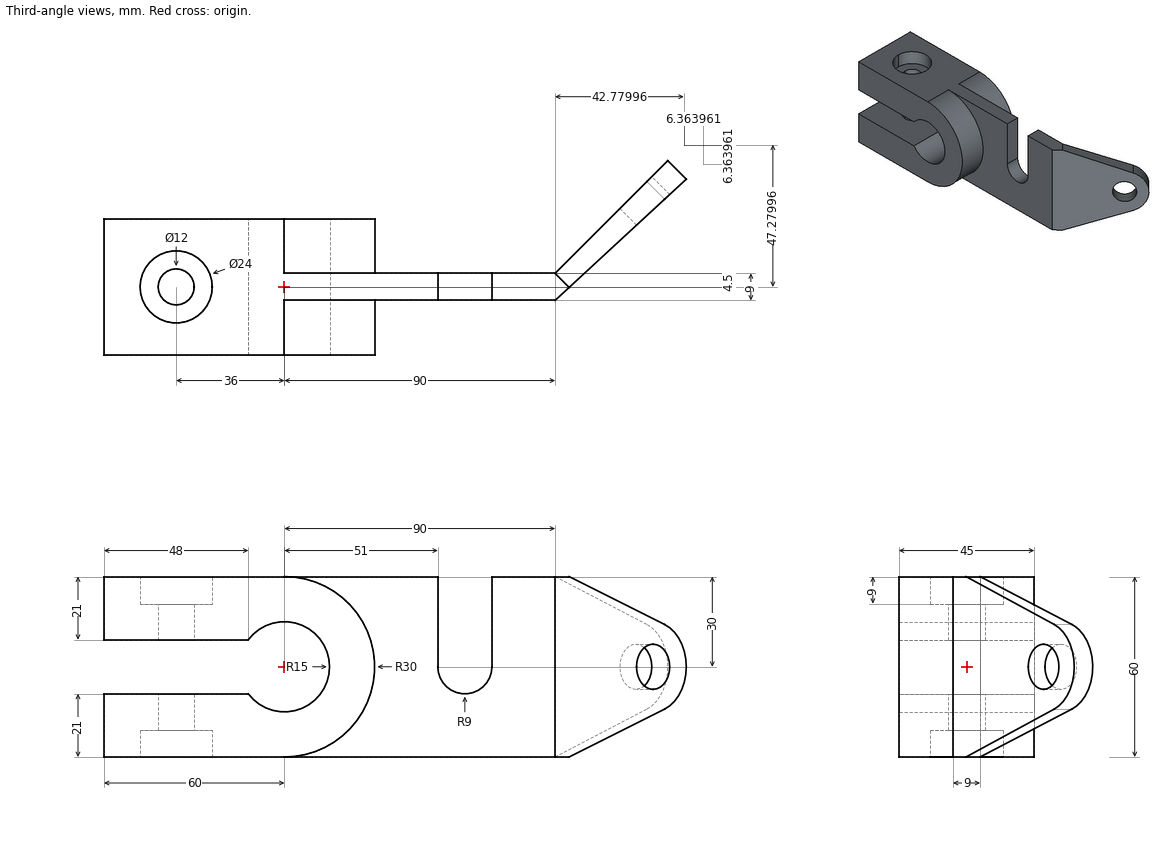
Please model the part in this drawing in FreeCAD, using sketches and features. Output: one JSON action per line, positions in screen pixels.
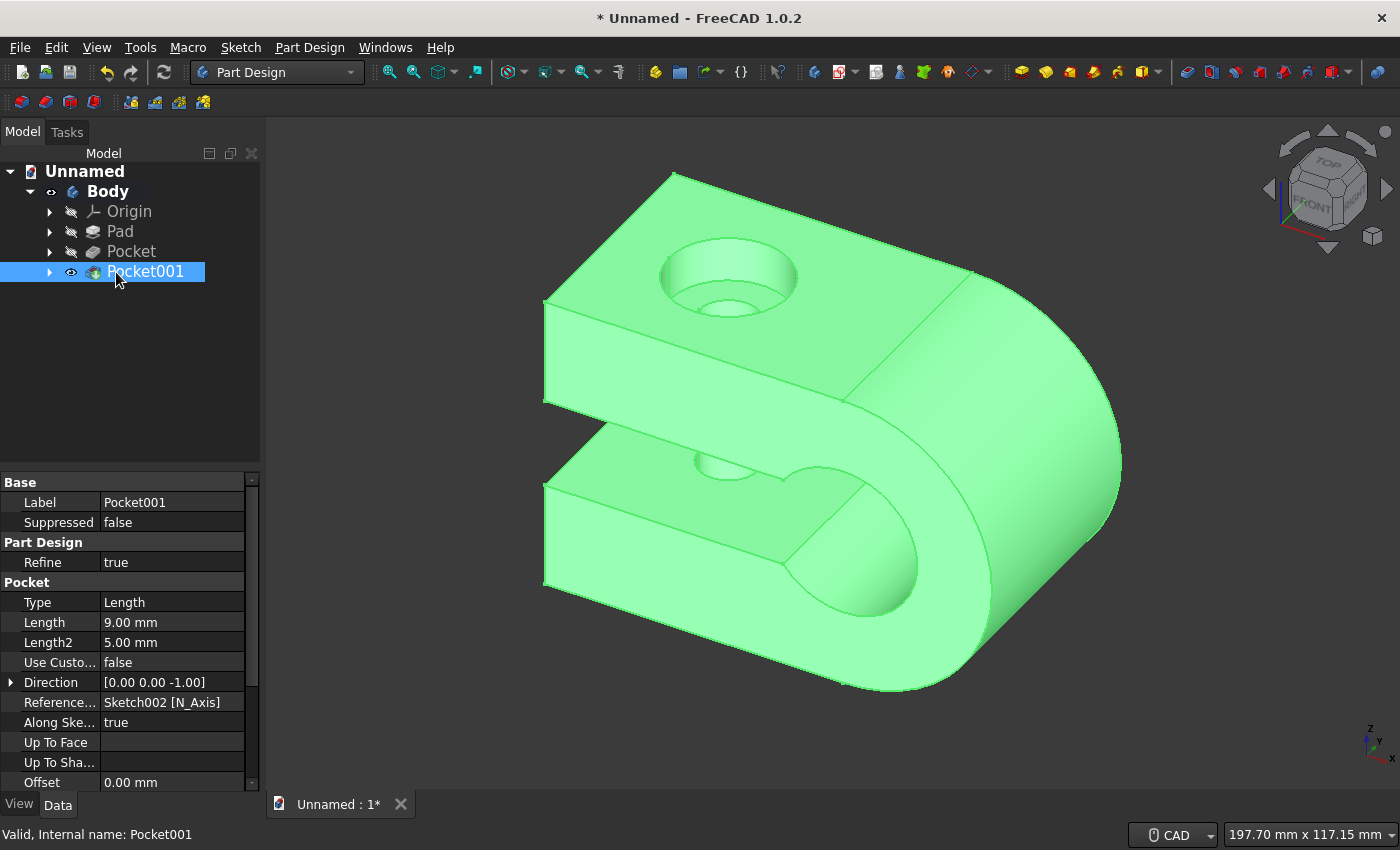
{"action": "left_click", "coordinate": [132, 102]}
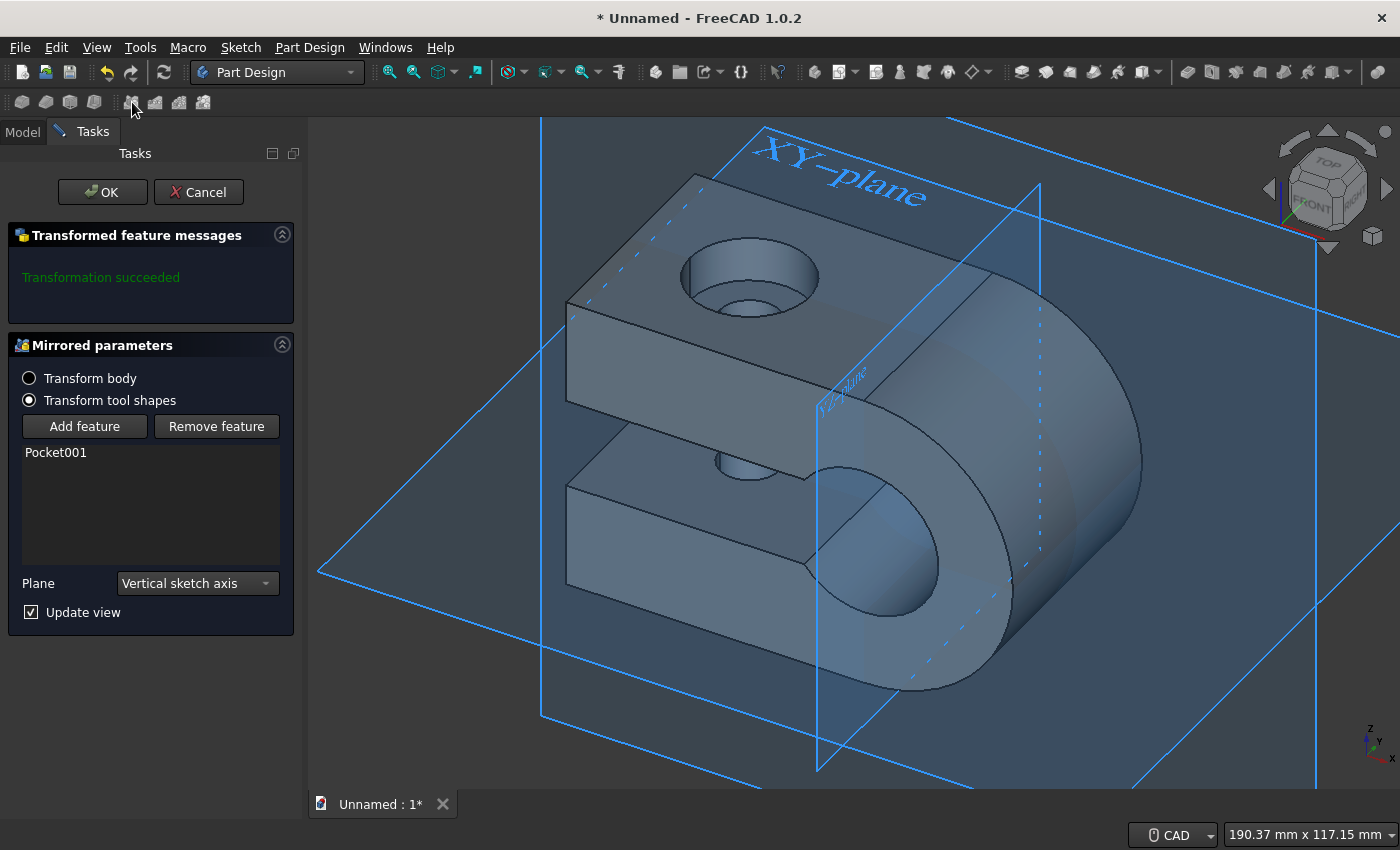
{"action": "left_click", "coordinate": [198, 584]}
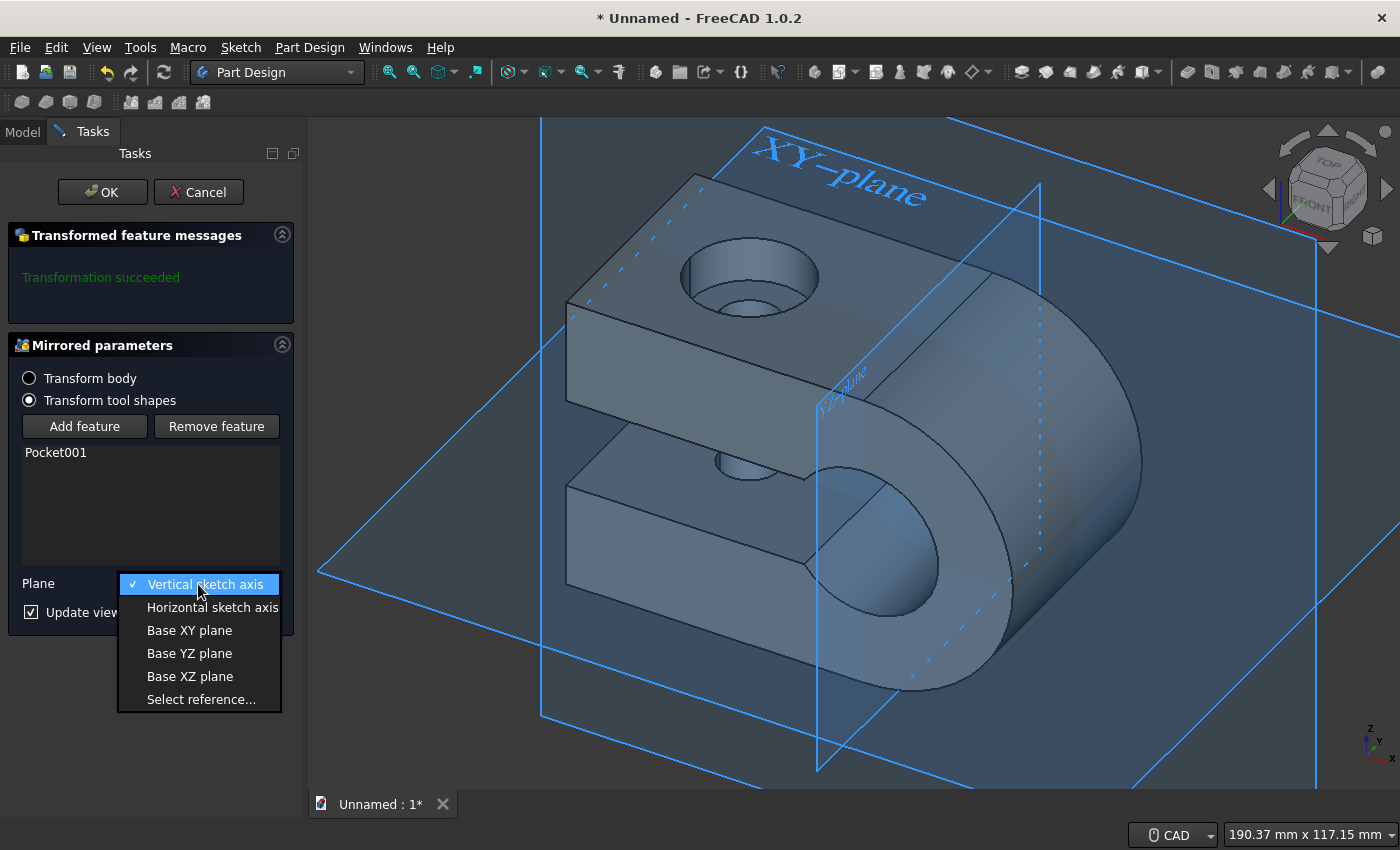
{"action": "left_click", "coordinate": [198, 630]}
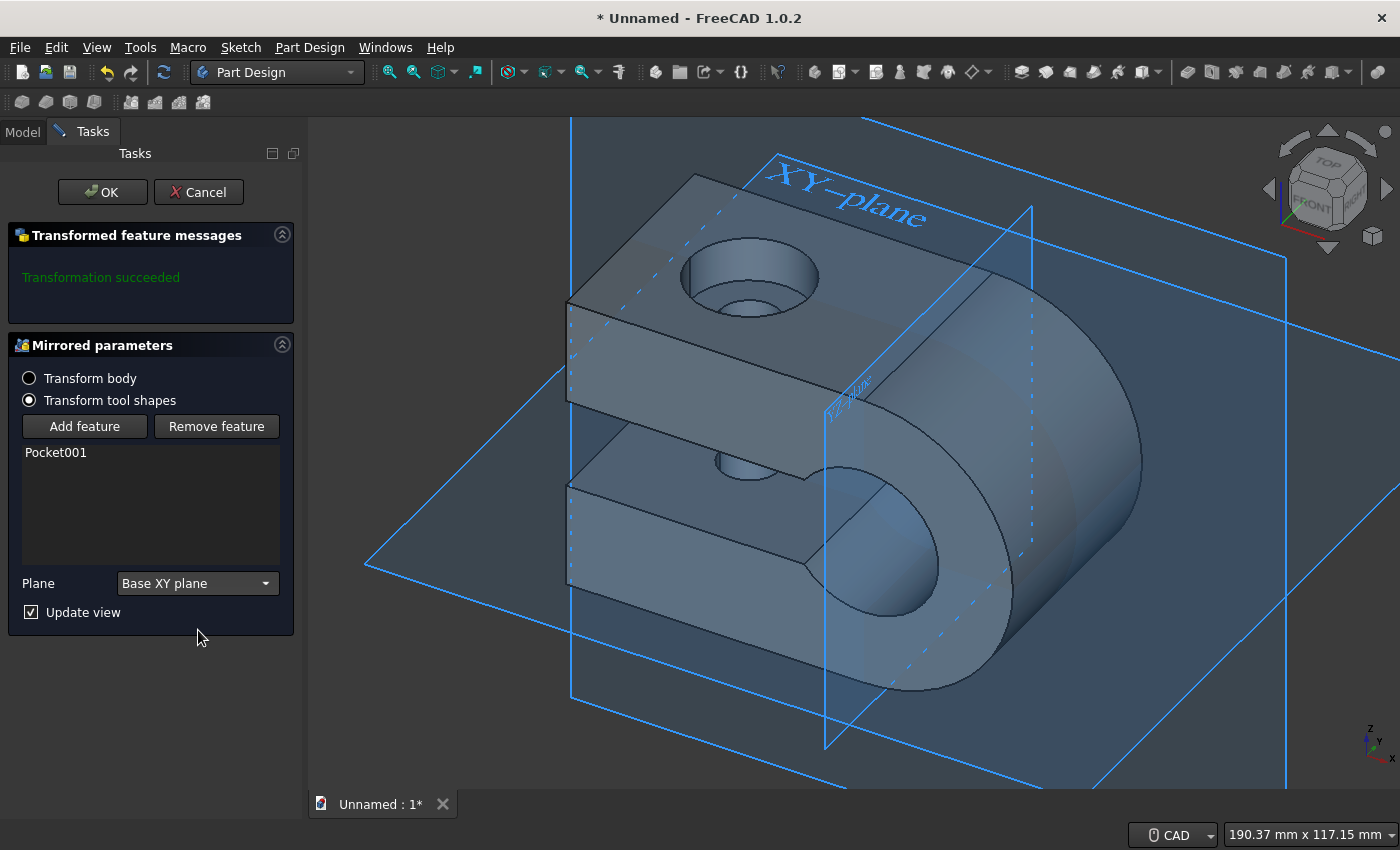
{"action": "left_click", "coordinate": [103, 192]}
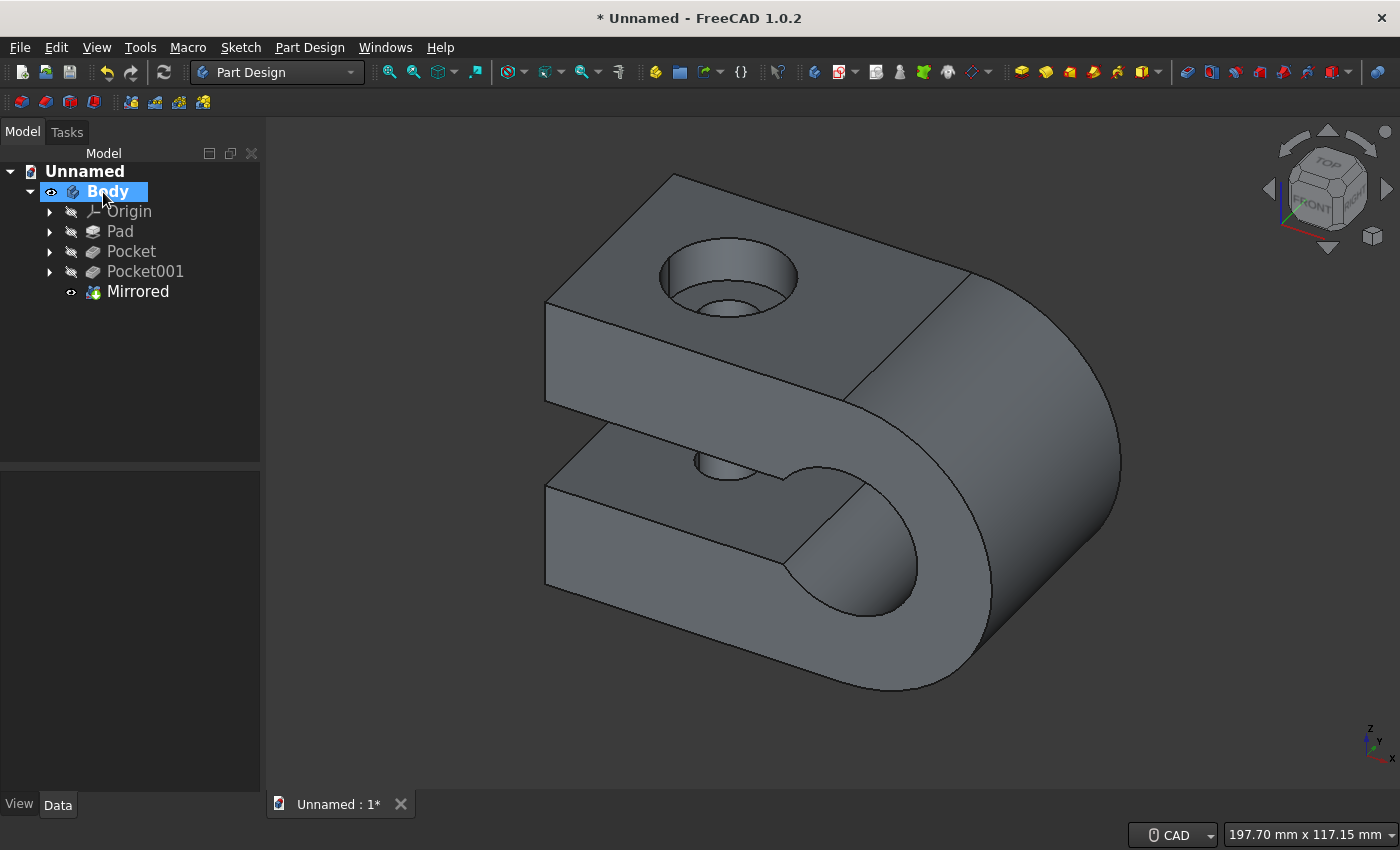
{"action": "left_click", "coordinate": [840, 72]}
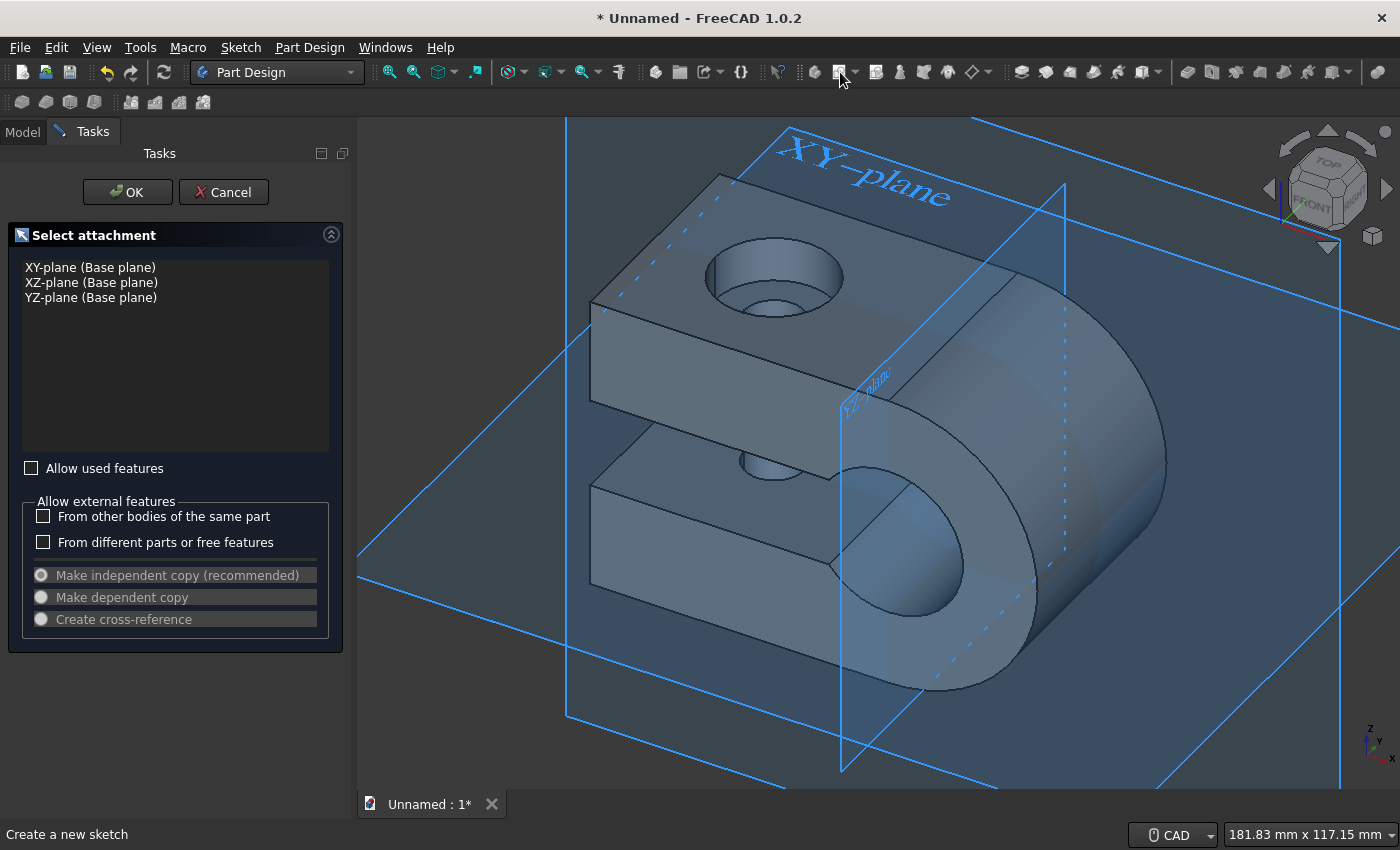
{"action": "left_click", "coordinate": [82, 282]}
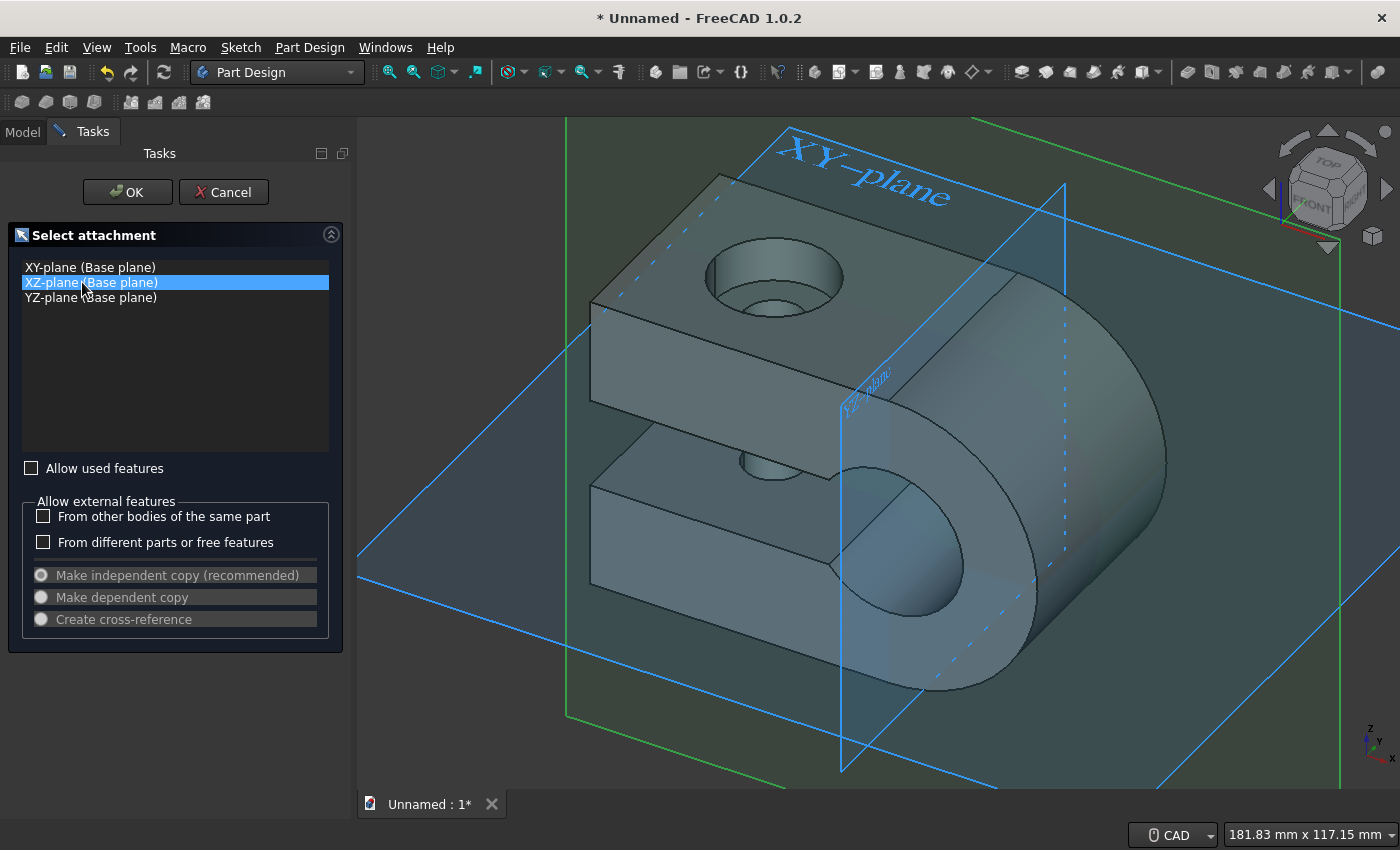
{"action": "left_click", "coordinate": [128, 192]}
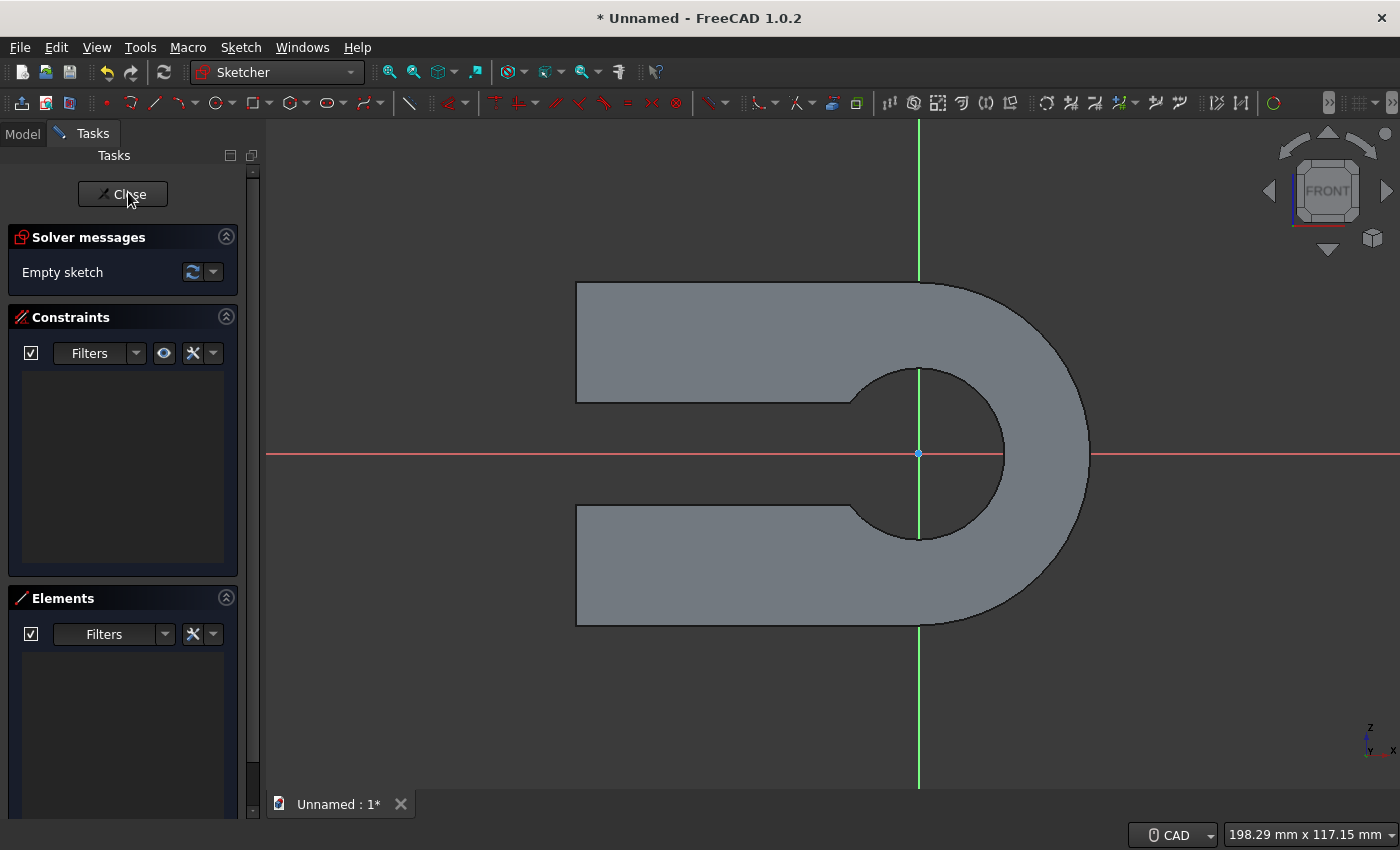
{"action": "key", "text": "q s"}